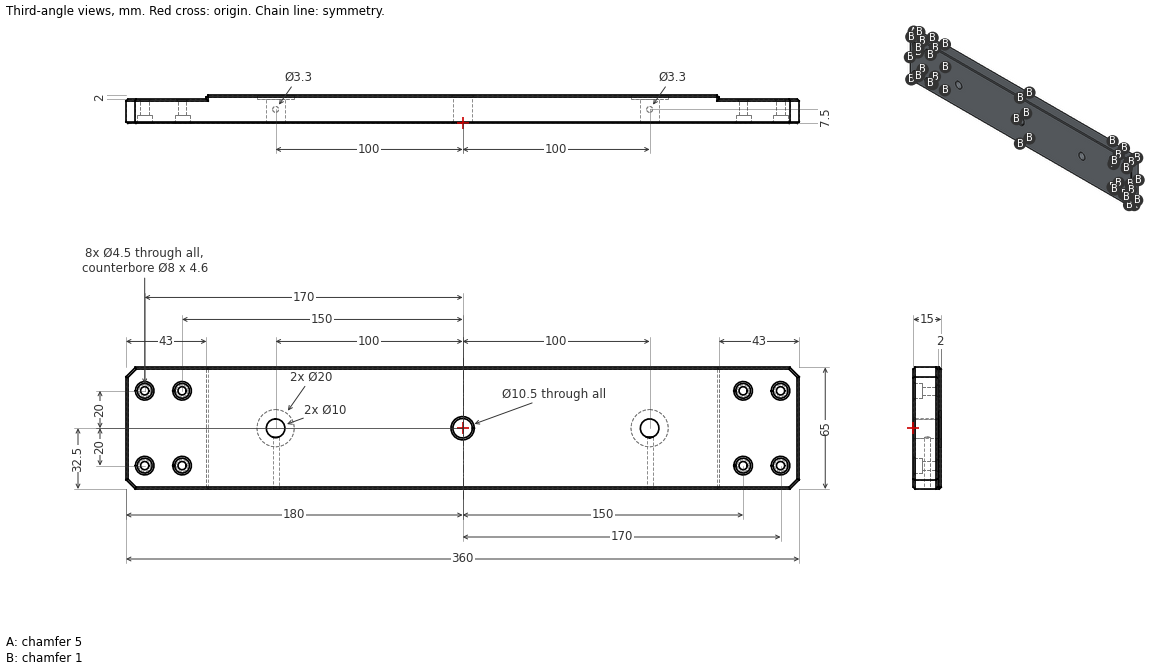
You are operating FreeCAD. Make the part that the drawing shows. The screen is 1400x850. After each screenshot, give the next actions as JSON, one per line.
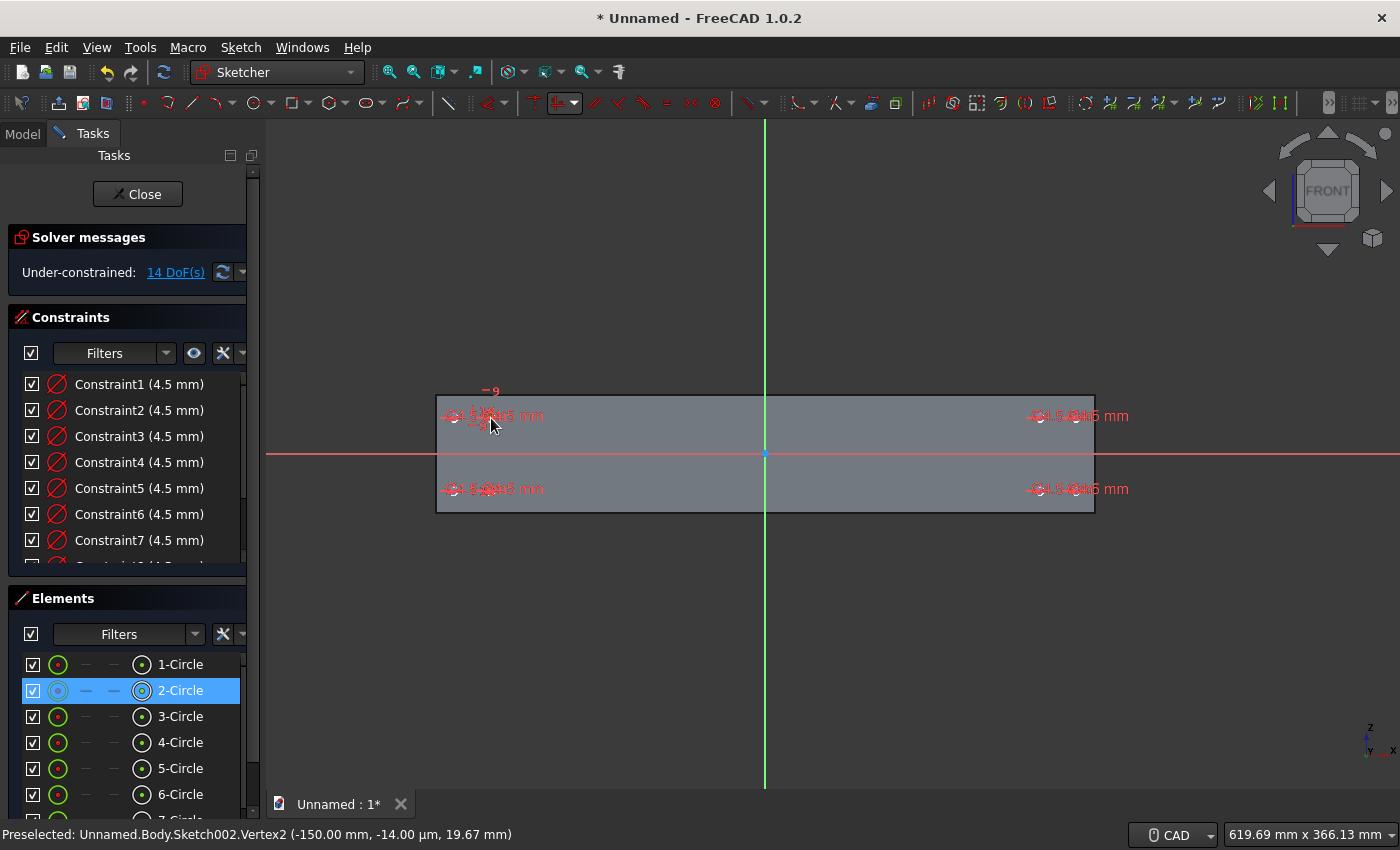
{"action": "scroll", "coordinate": [491, 491], "scroll_direction": "up", "scroll_amount": 4}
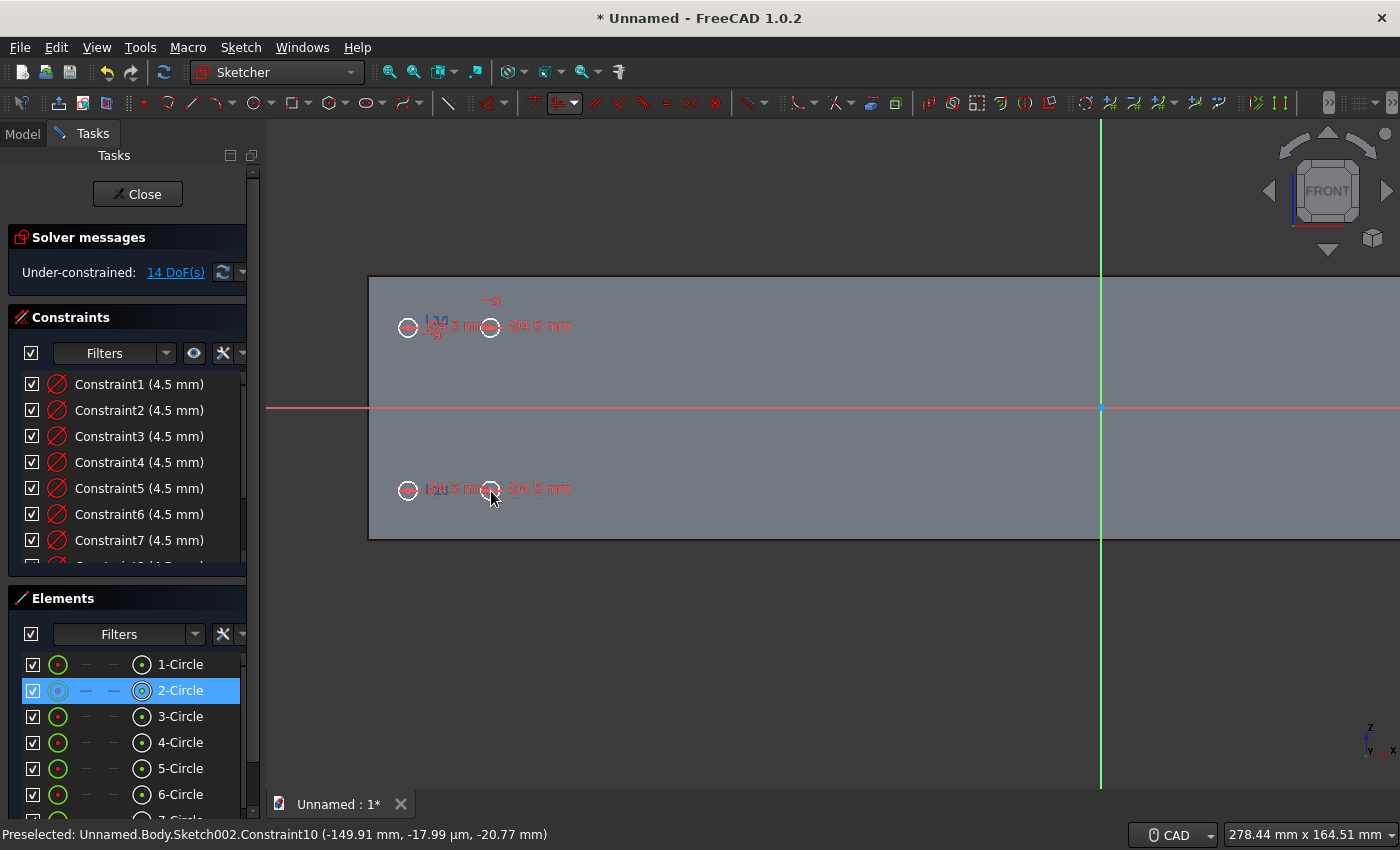
{"action": "left_click", "coordinate": [490, 491]}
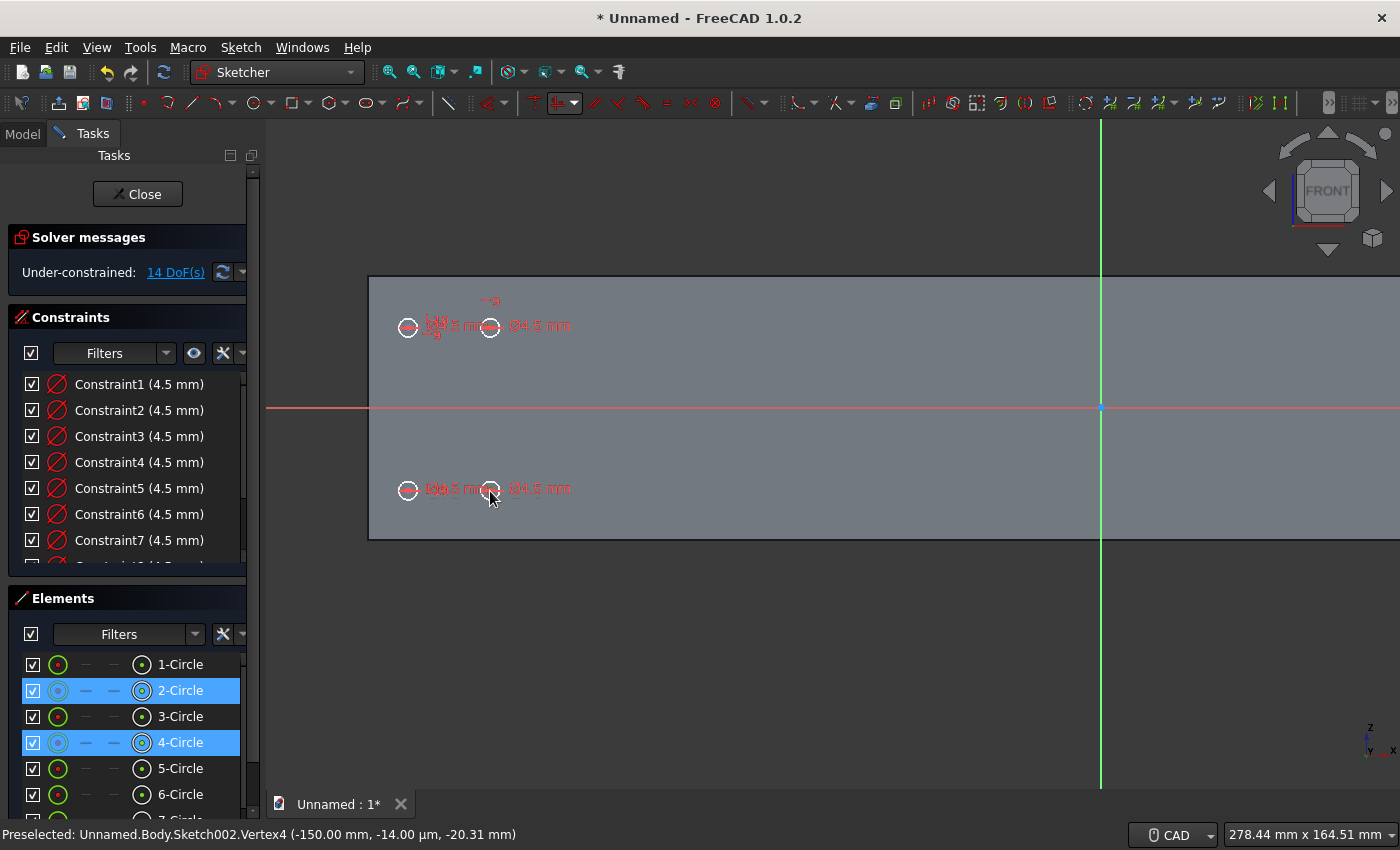
{"action": "key", "text": "v"}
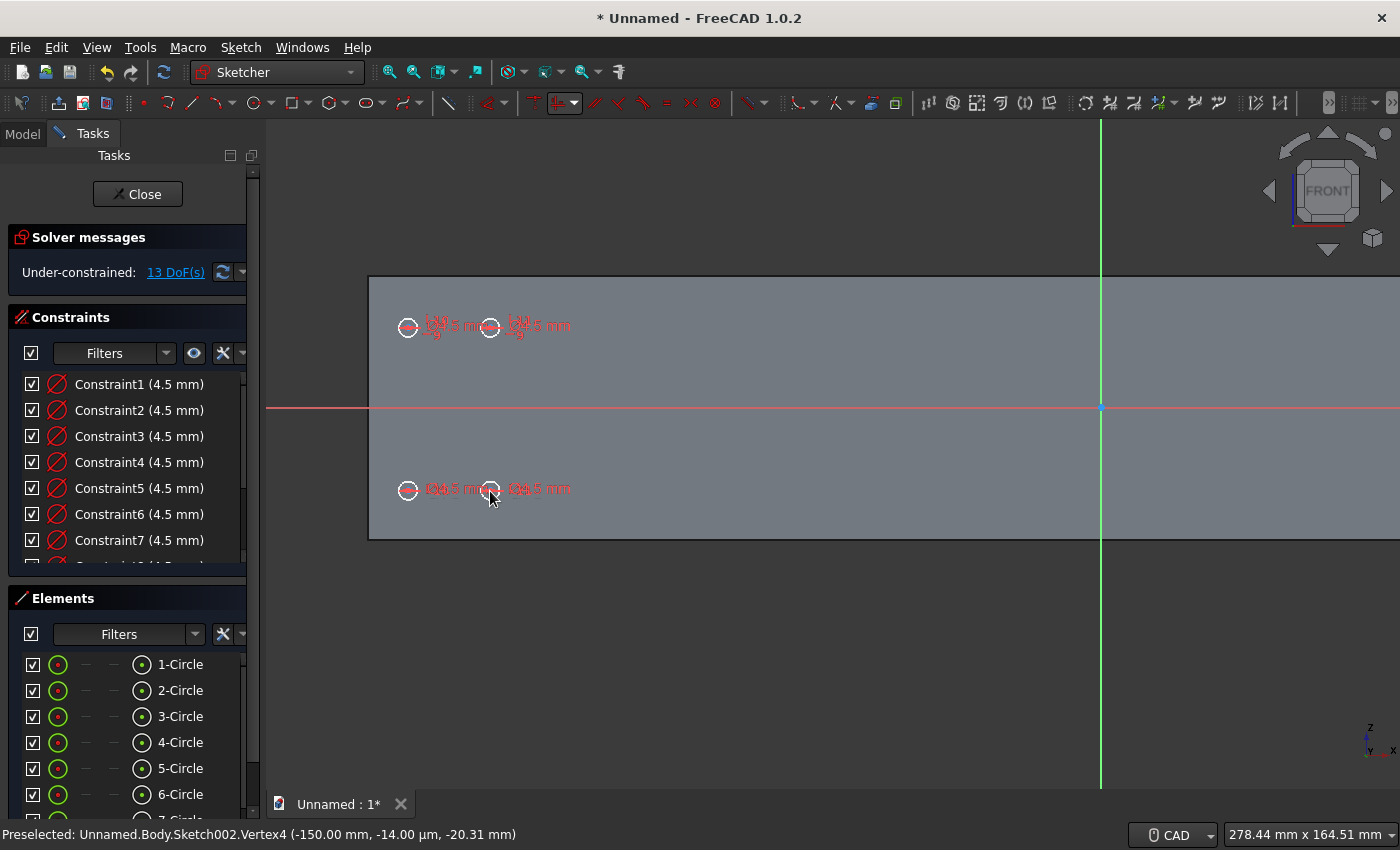
{"action": "left_click", "coordinate": [408, 491]}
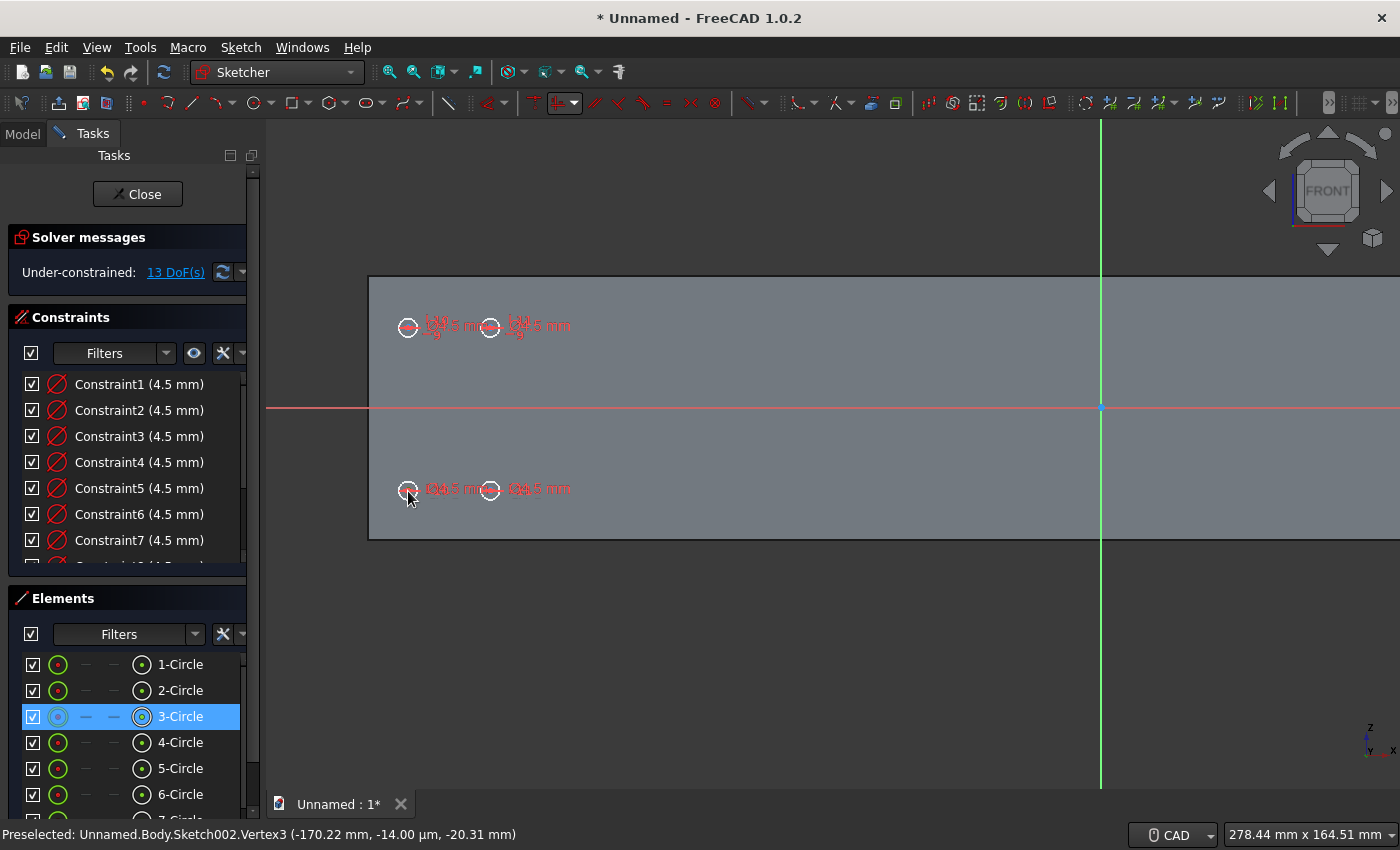
{"action": "left_click", "coordinate": [490, 491]}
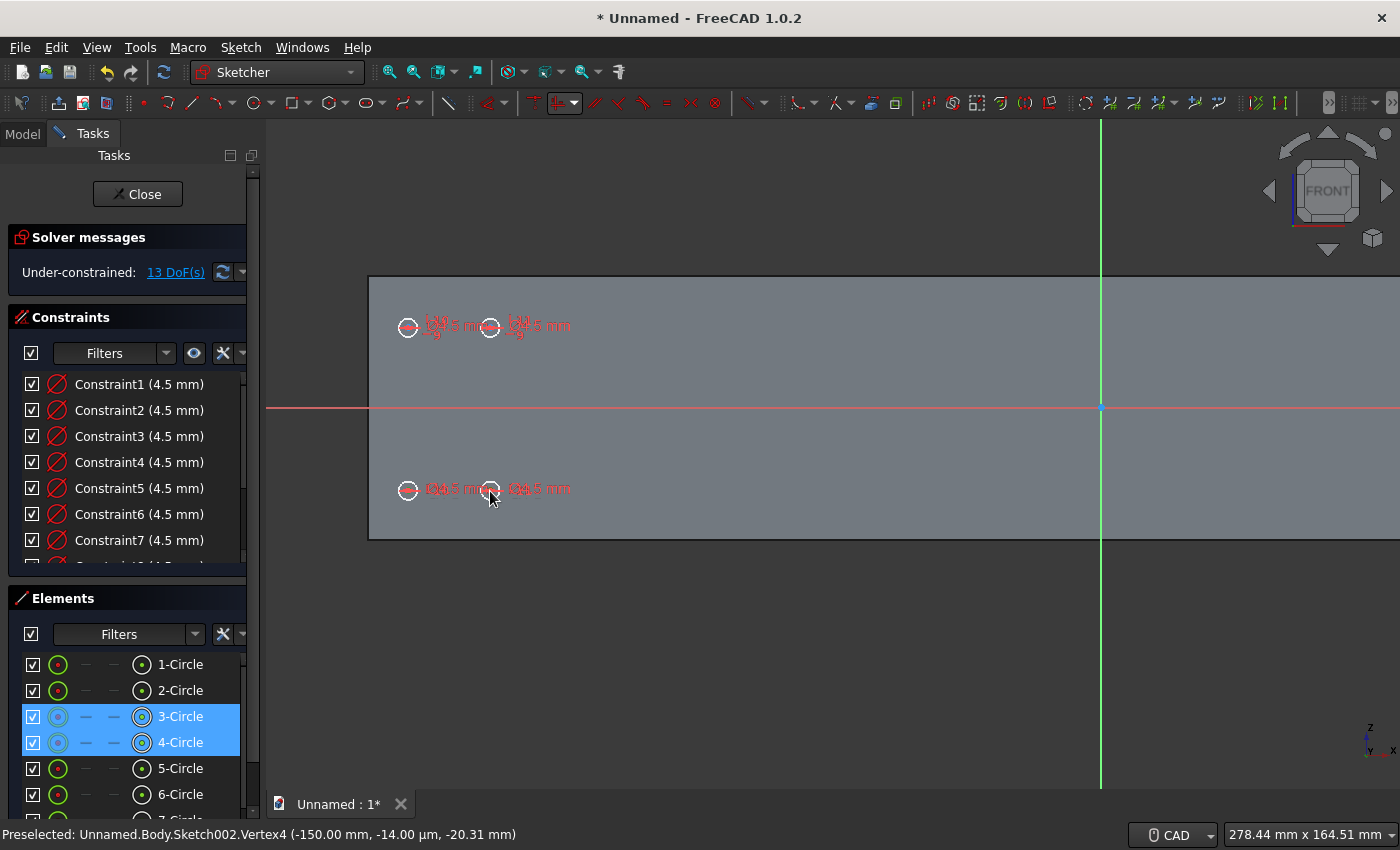
{"action": "key", "text": "h"}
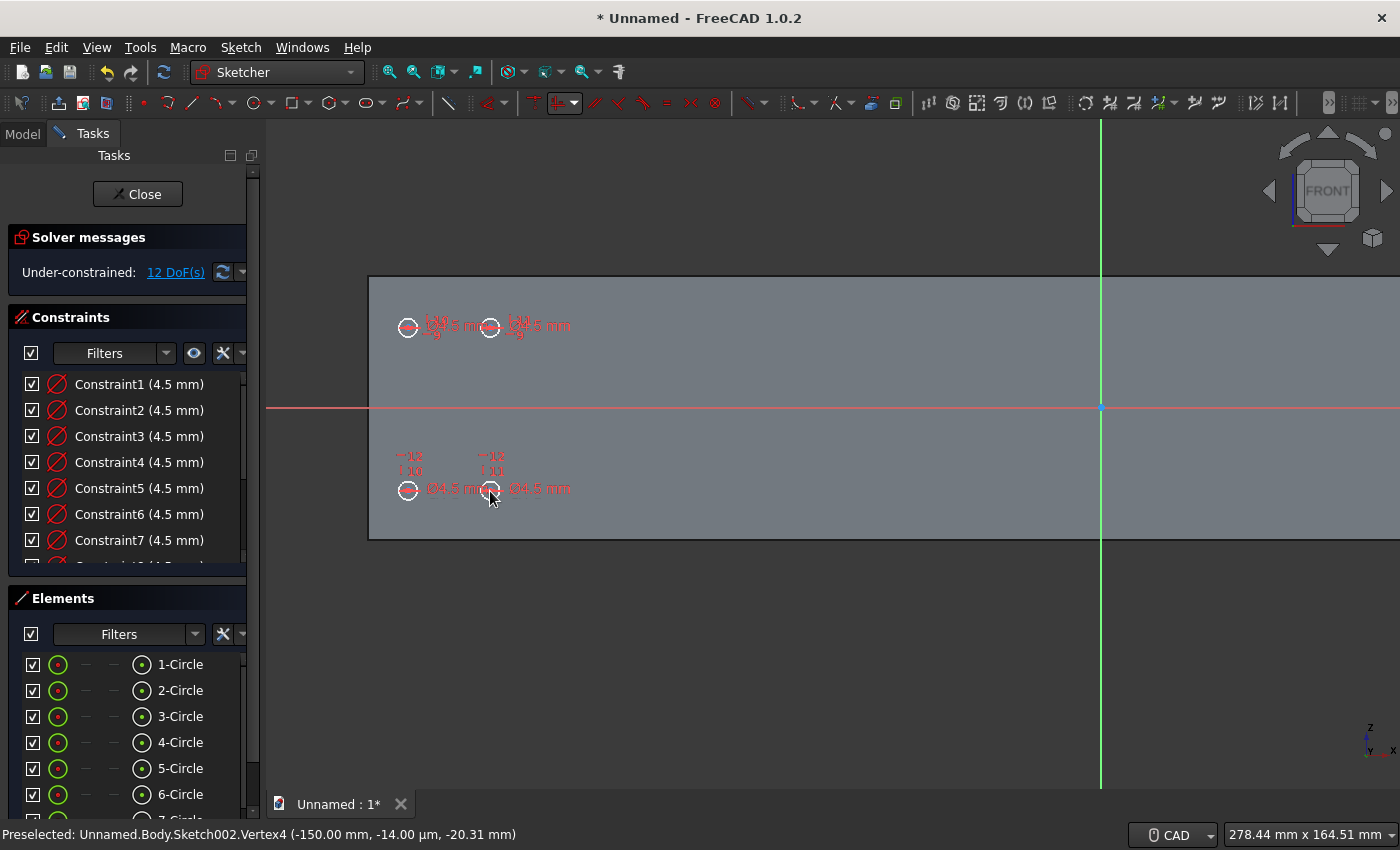
{"action": "left_click", "coordinate": [490, 491]}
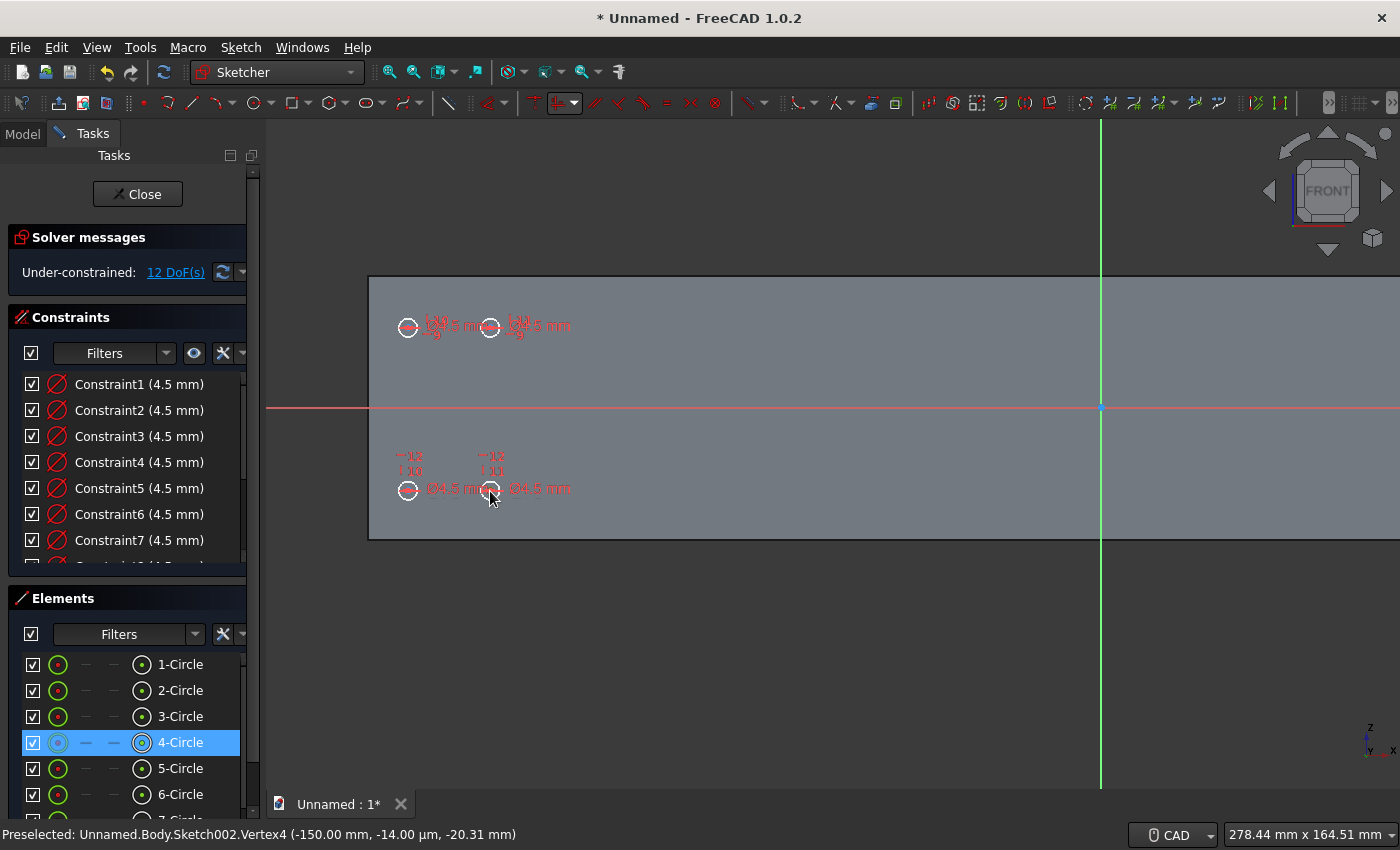
{"action": "scroll", "coordinate": [490, 492], "scroll_direction": "down", "scroll_amount": 4}